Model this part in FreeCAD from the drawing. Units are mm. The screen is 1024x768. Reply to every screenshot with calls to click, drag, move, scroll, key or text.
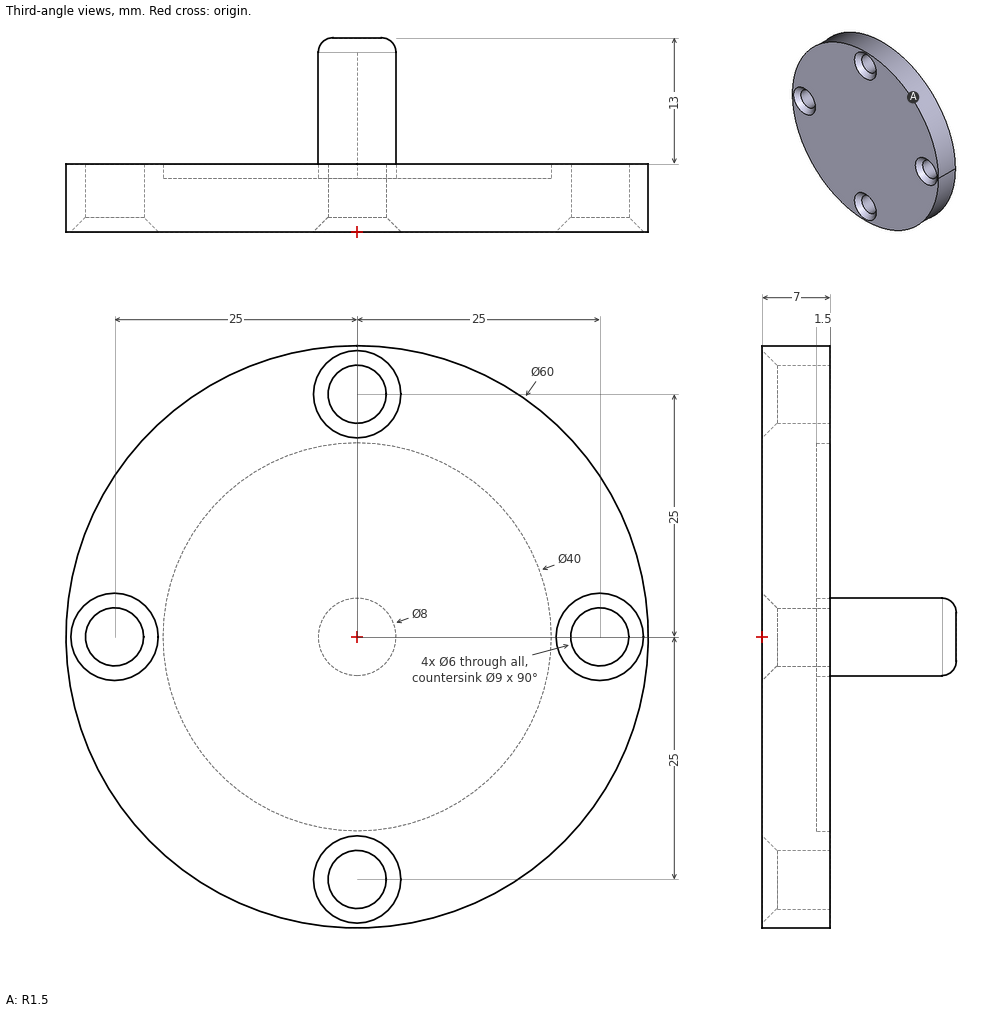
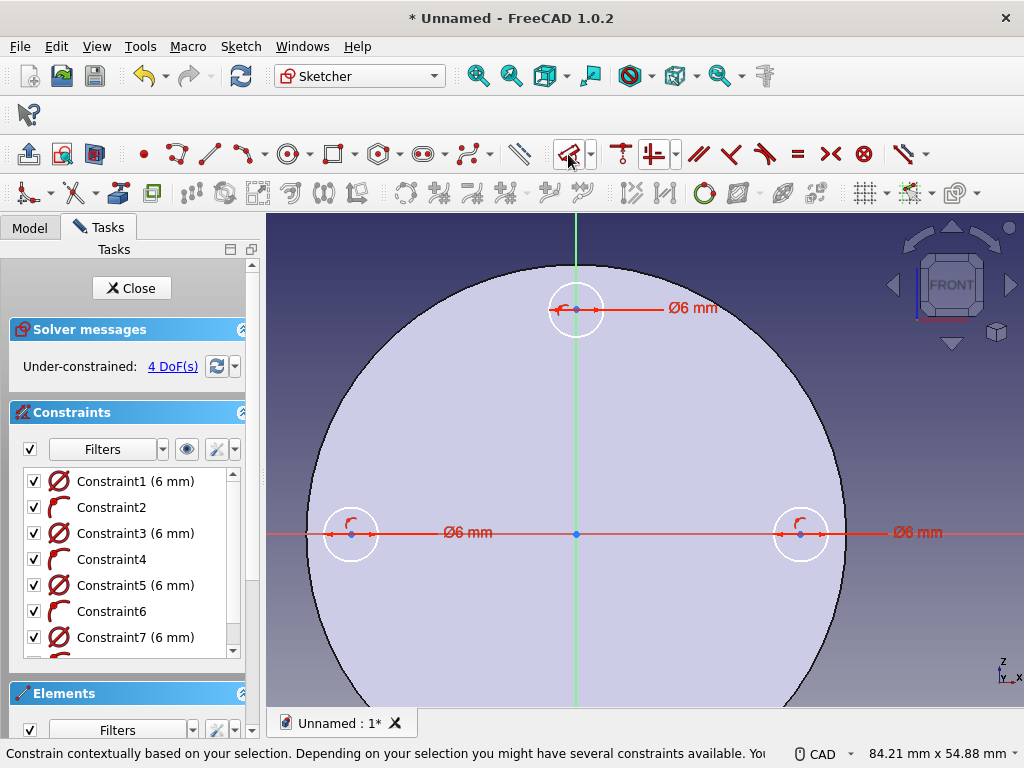
click(801, 534)
click(689, 568)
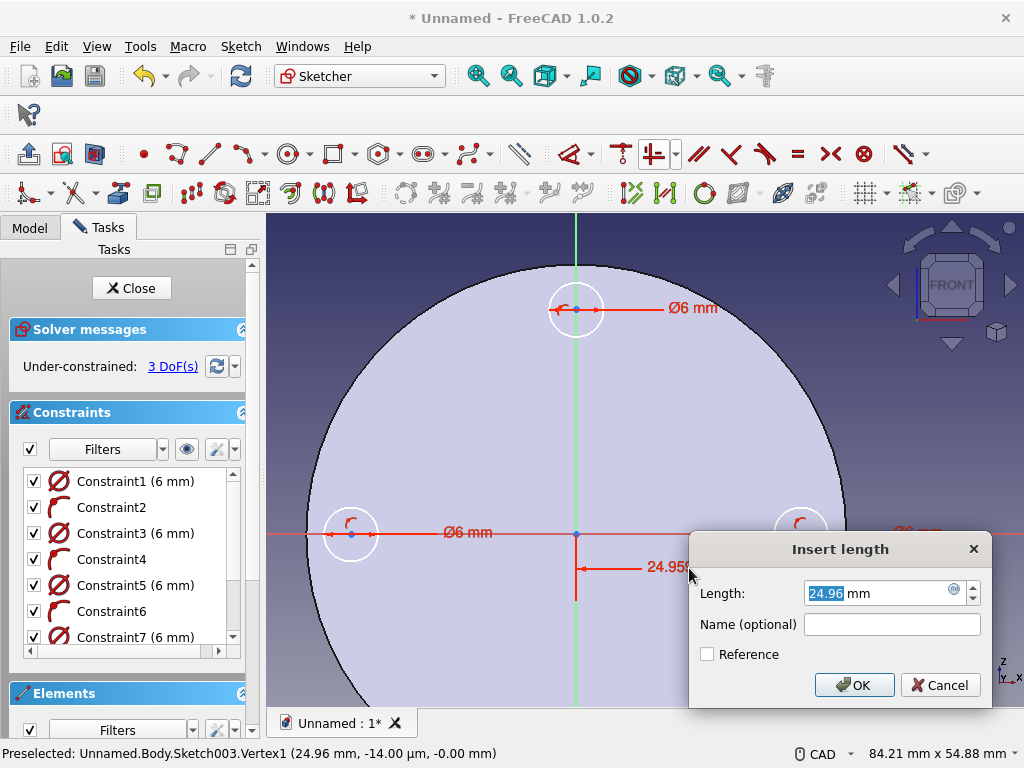
text(25)
key(Return)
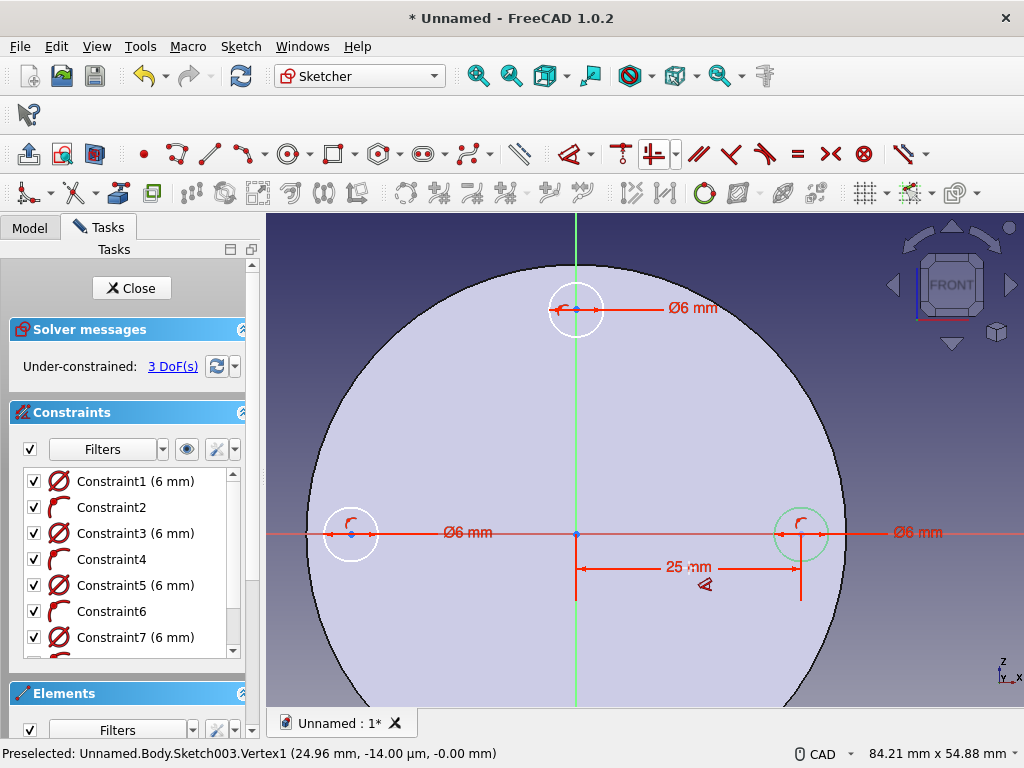
scroll(577, 309, down, 2)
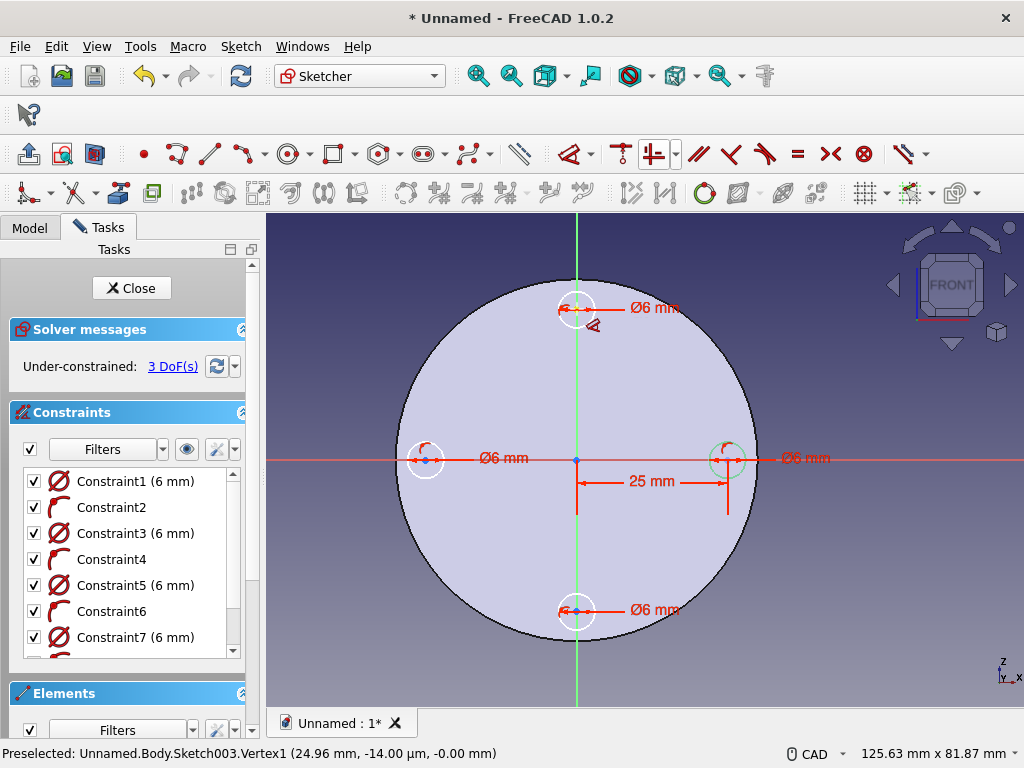
click(577, 612)
click(611, 536)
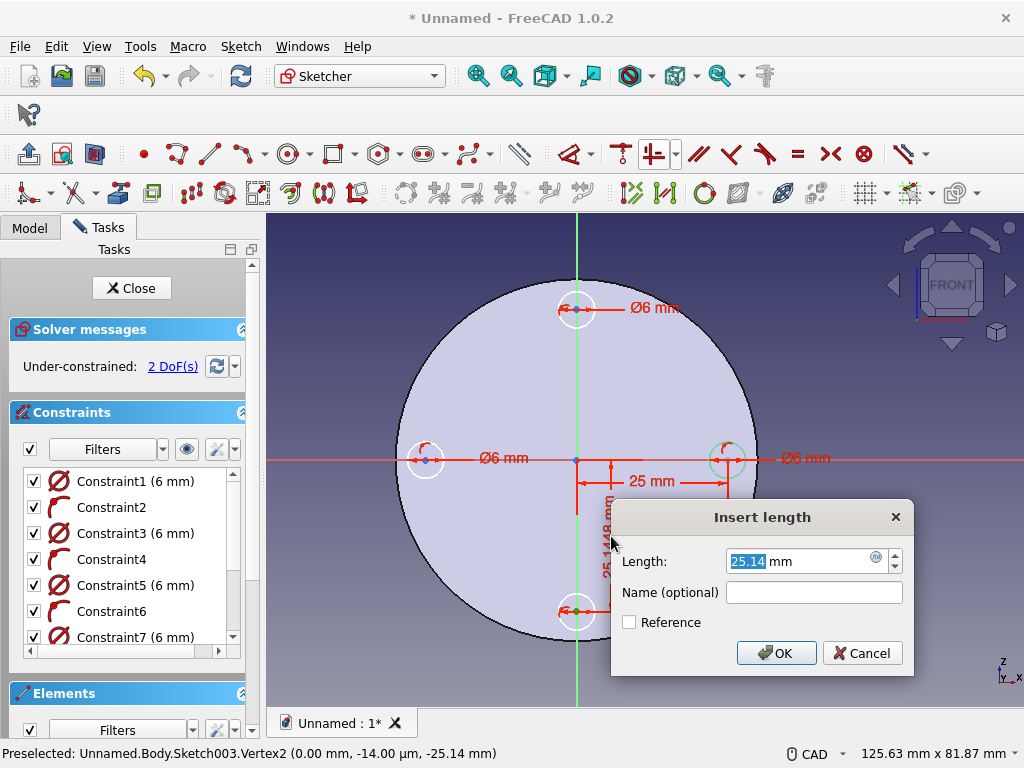
text(25)
key(Return)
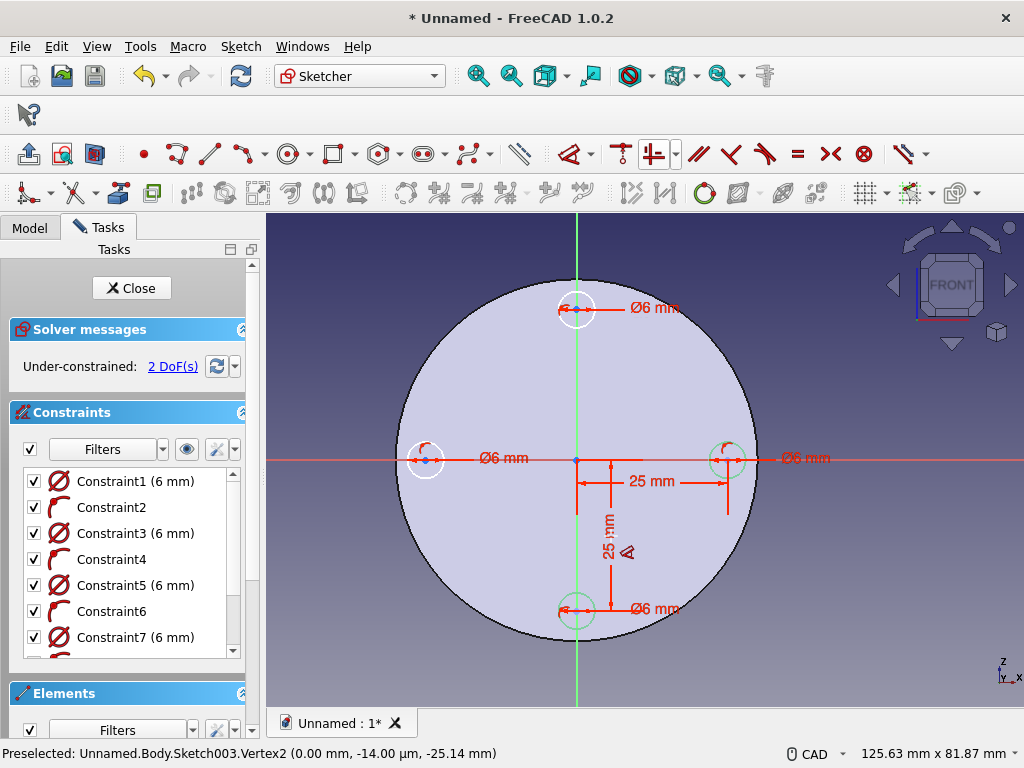
click(426, 460)
click(501, 494)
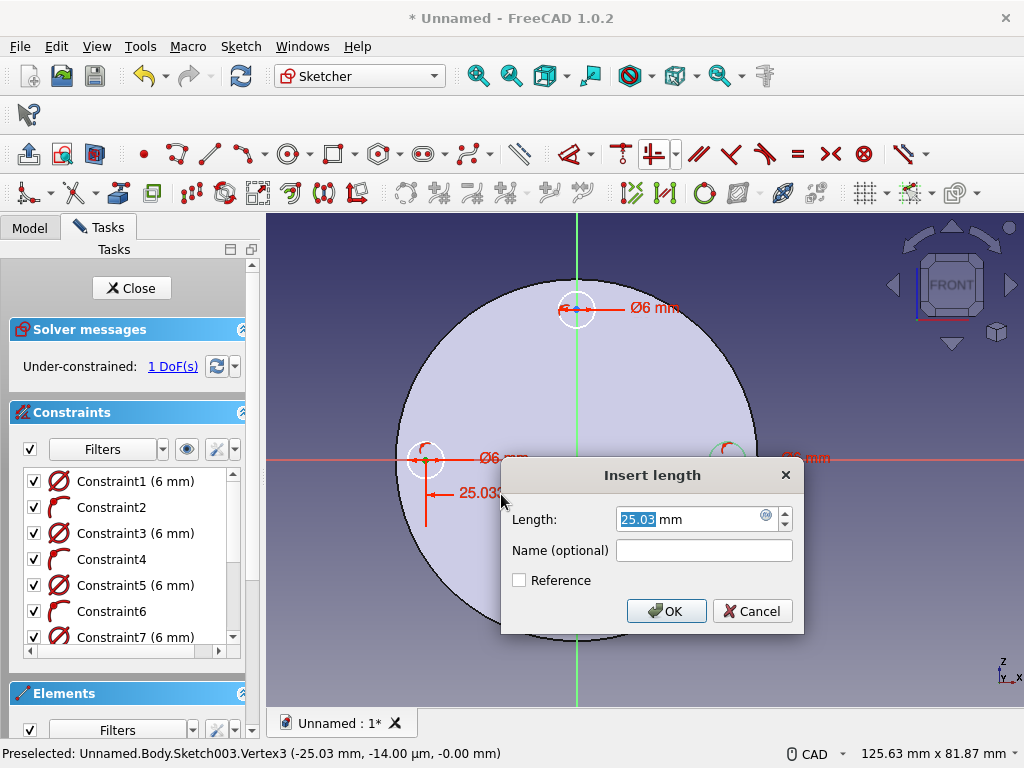
text(25)
key(Return)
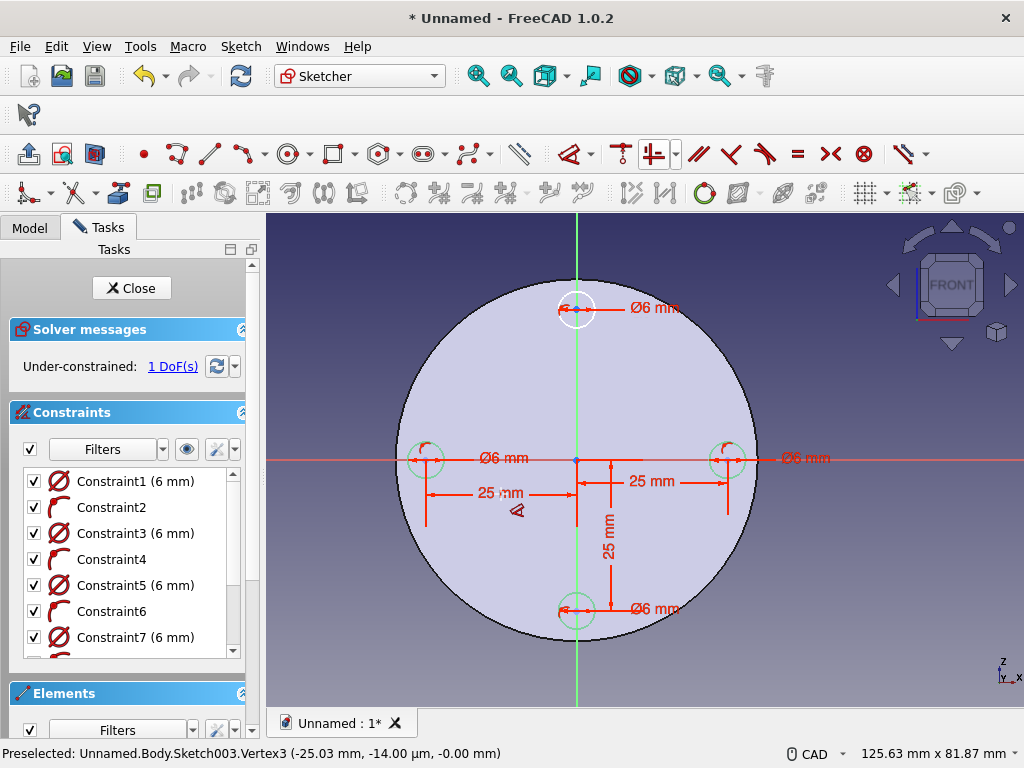
click(577, 310)
click(611, 385)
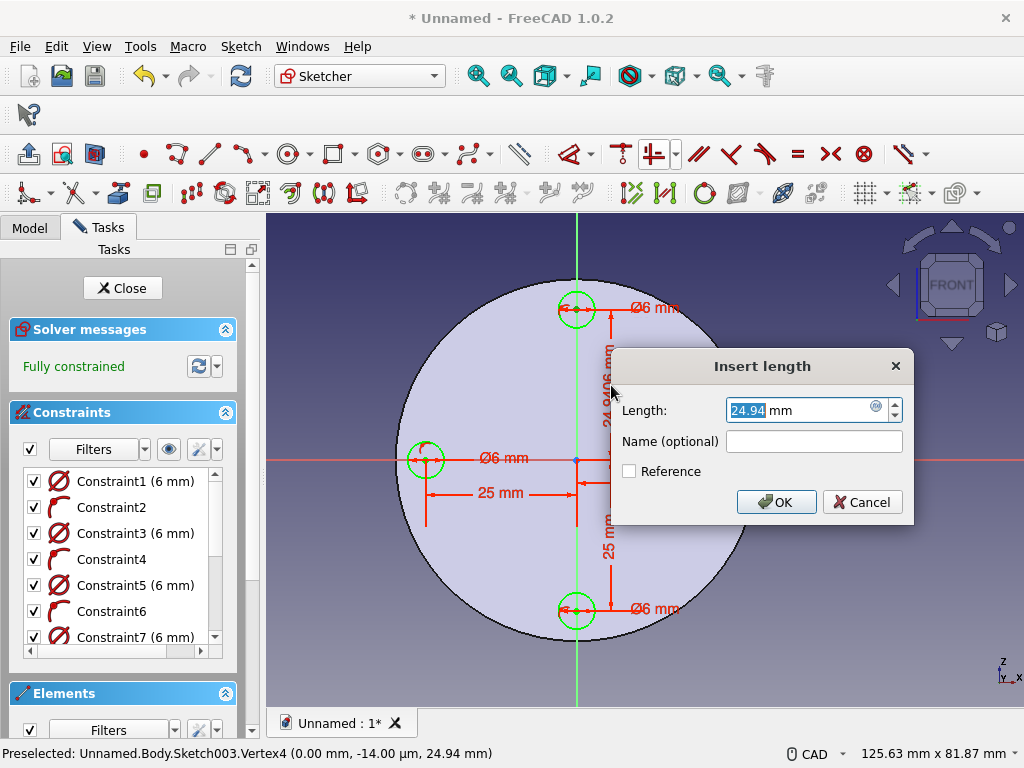
text(25)
key(Return)
key(Escape)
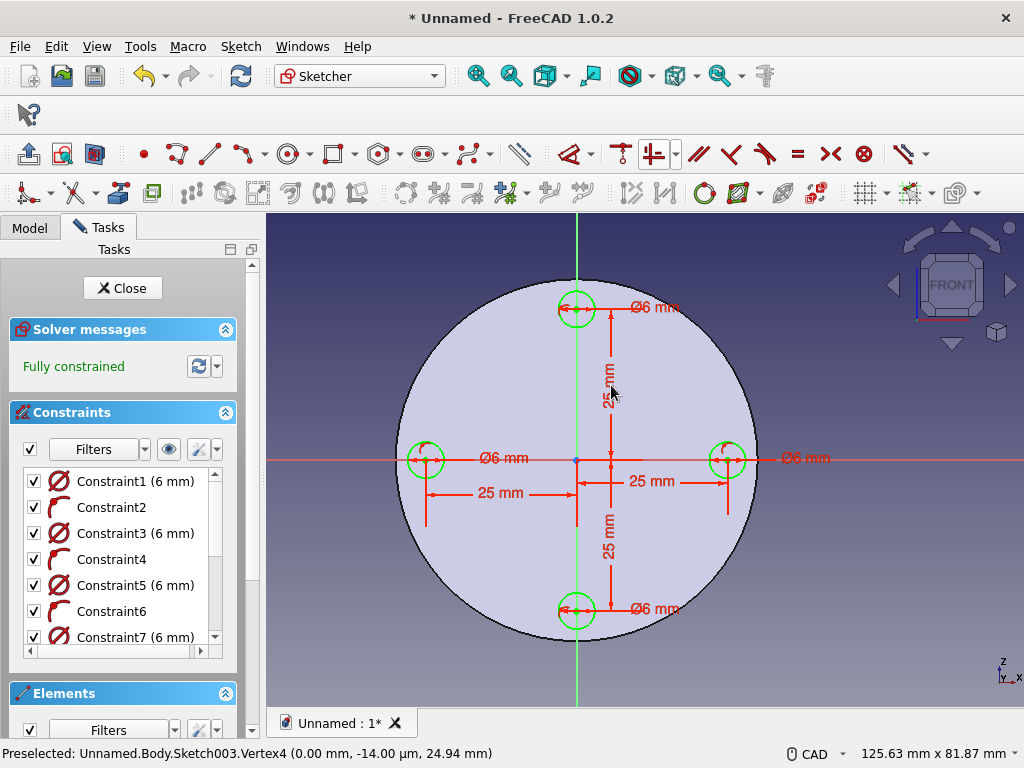
click(123, 288)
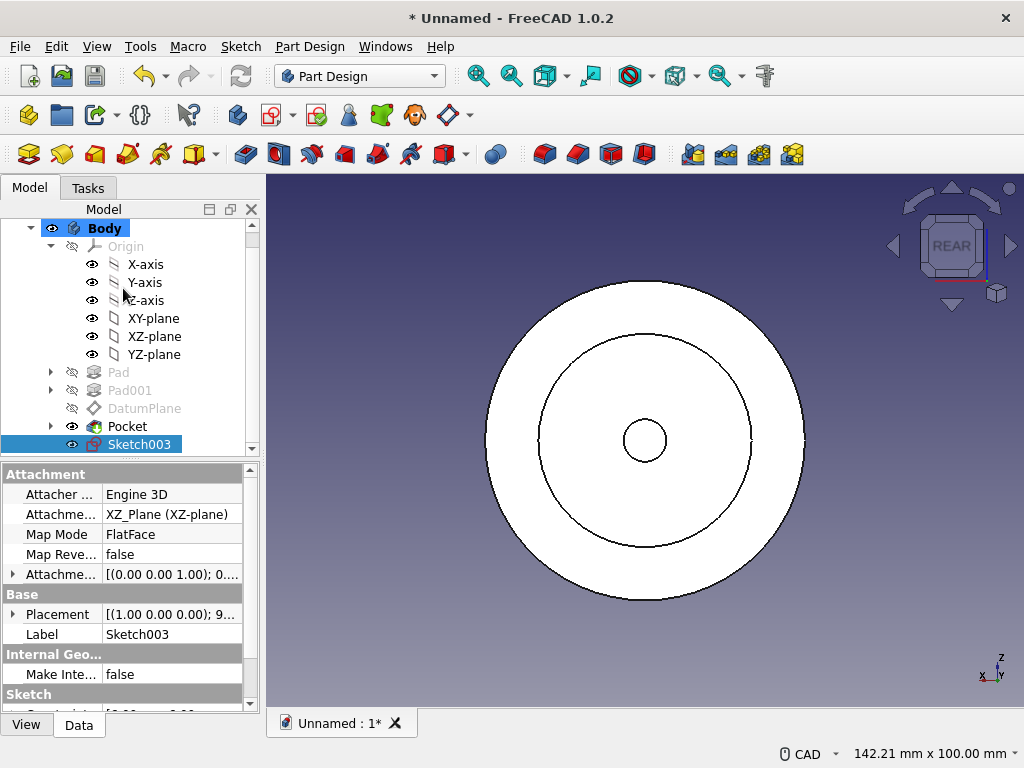
click(279, 154)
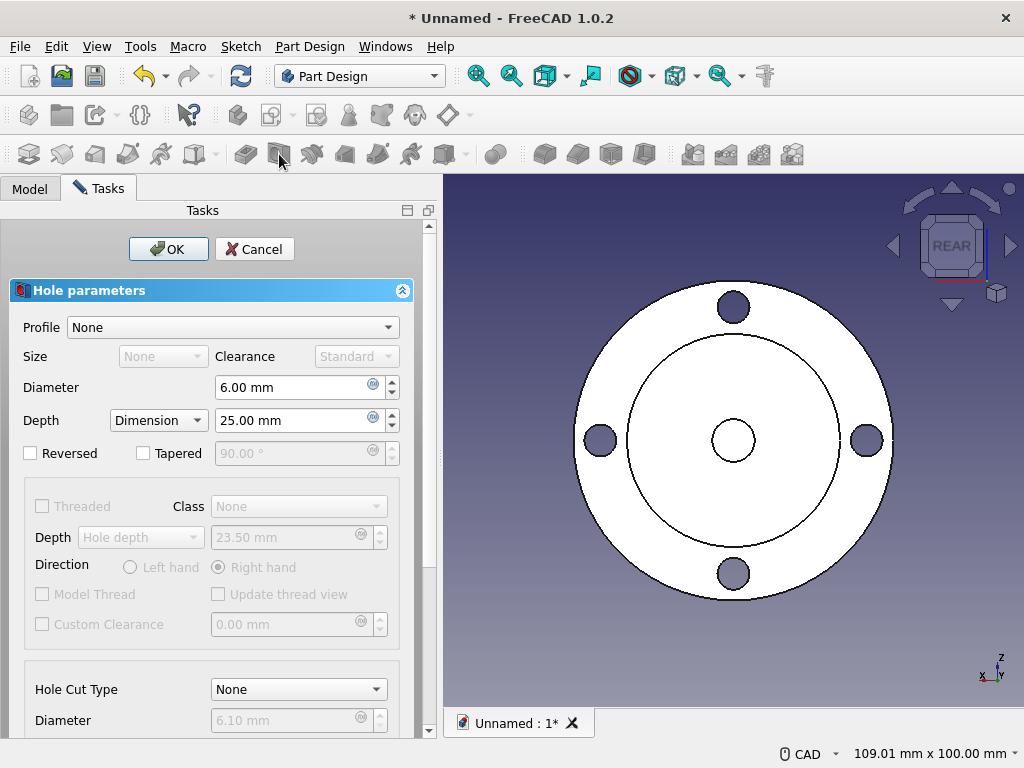
triple_click(300, 388)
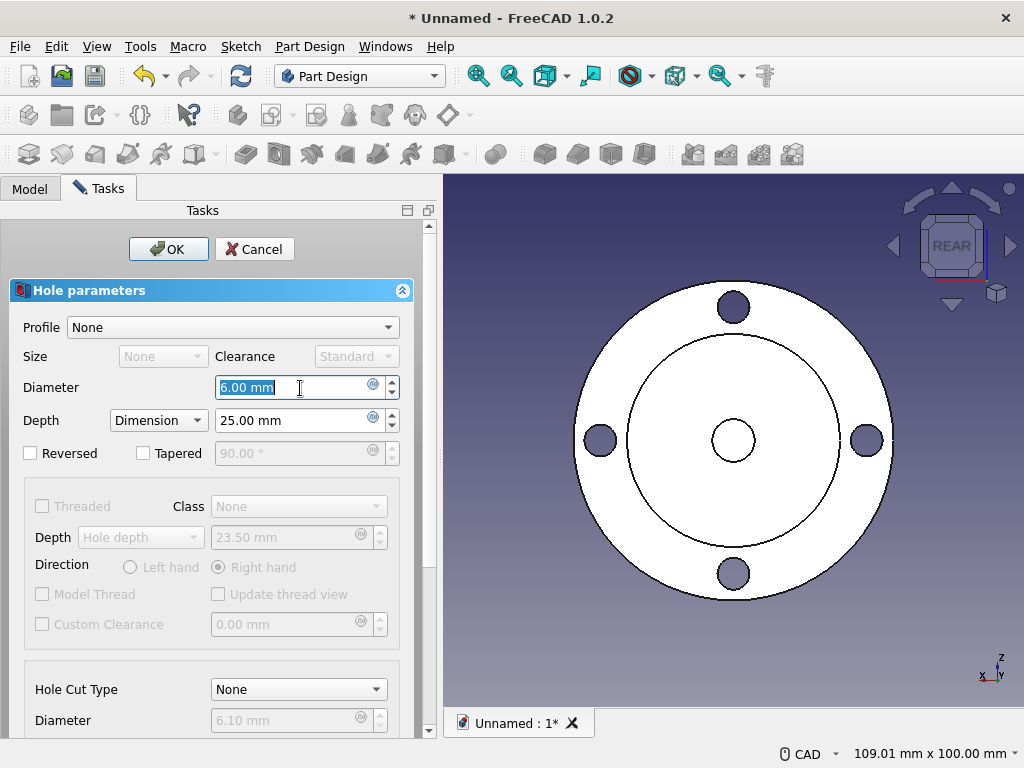
text(6)
key(Tab)